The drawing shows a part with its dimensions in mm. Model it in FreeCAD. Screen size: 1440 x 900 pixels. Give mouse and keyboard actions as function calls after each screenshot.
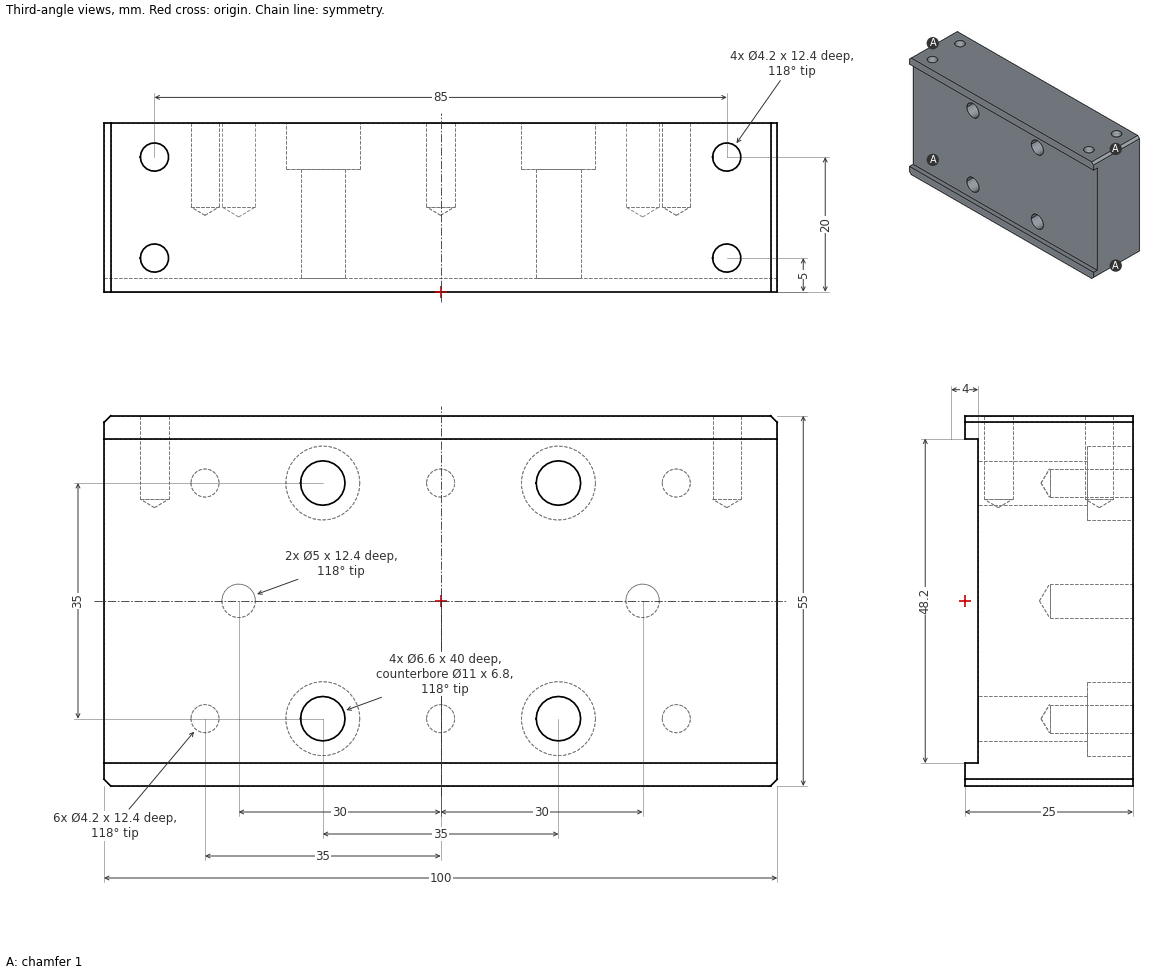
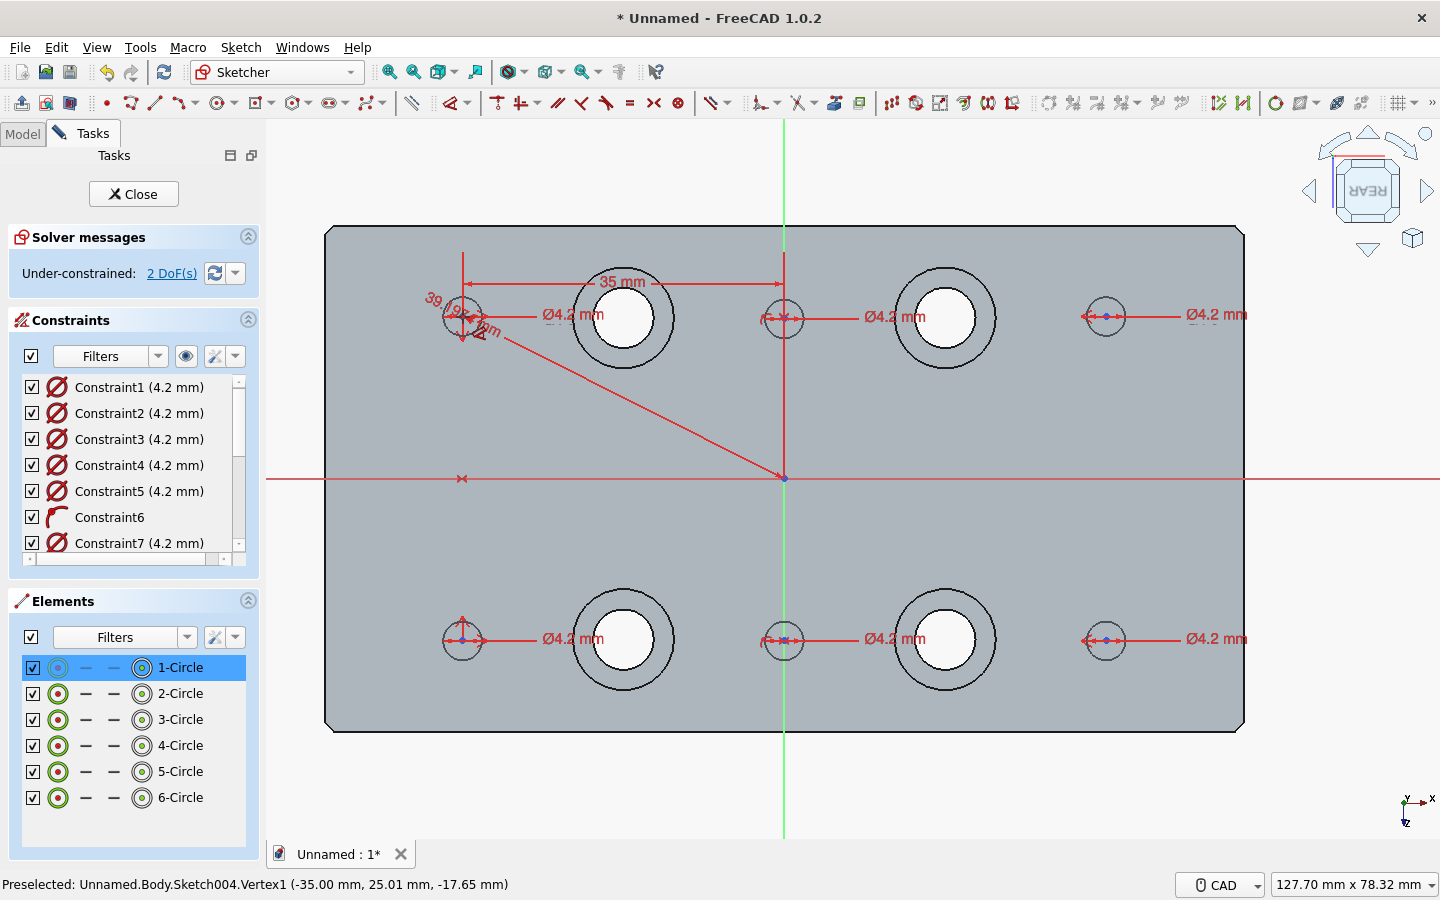
click(463, 641)
click(429, 404)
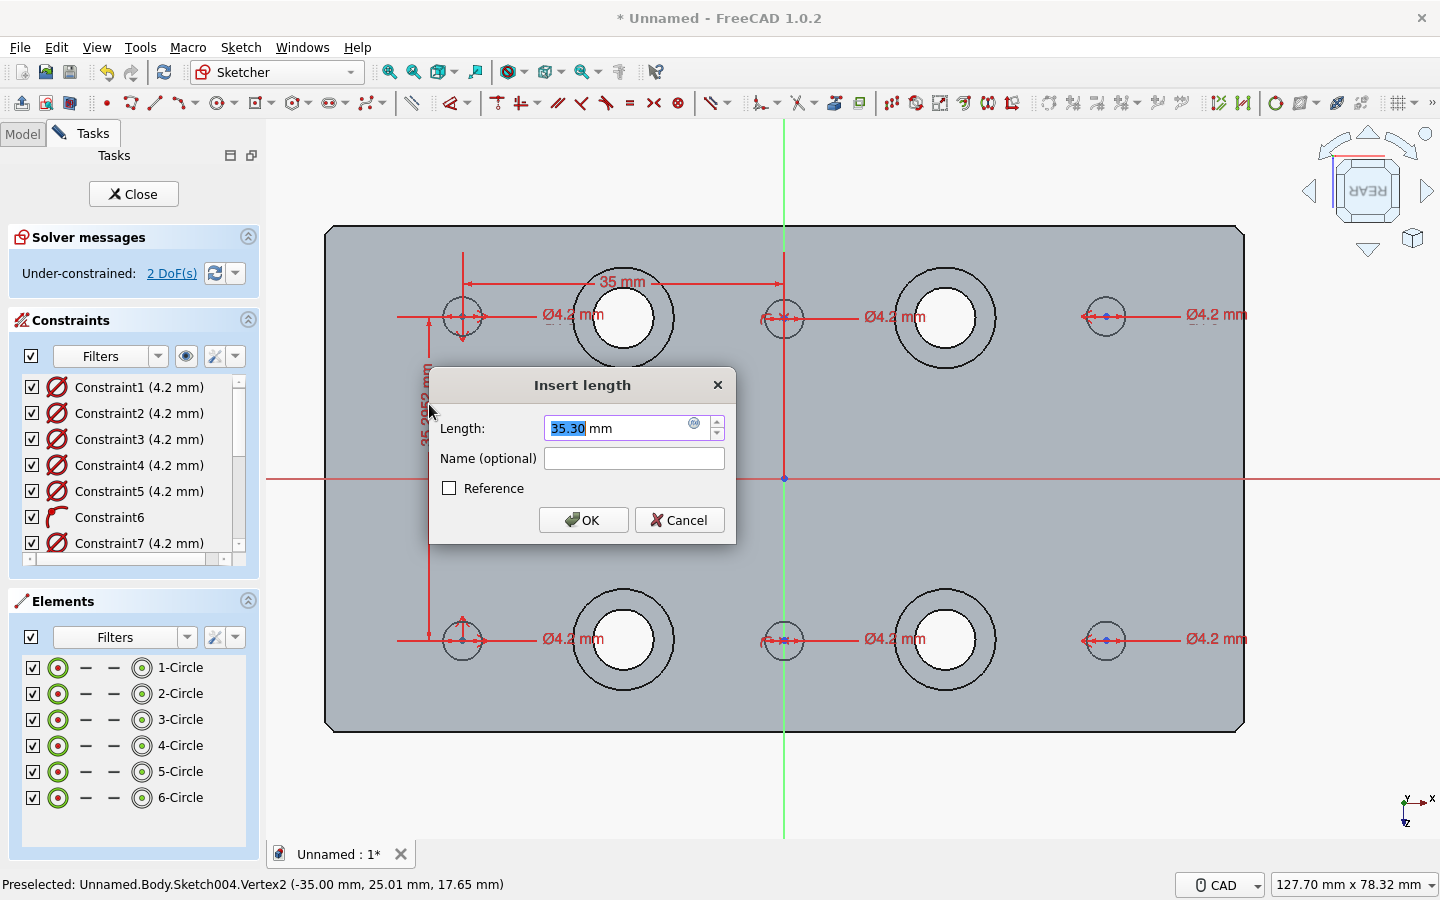
text(35)
key(Return)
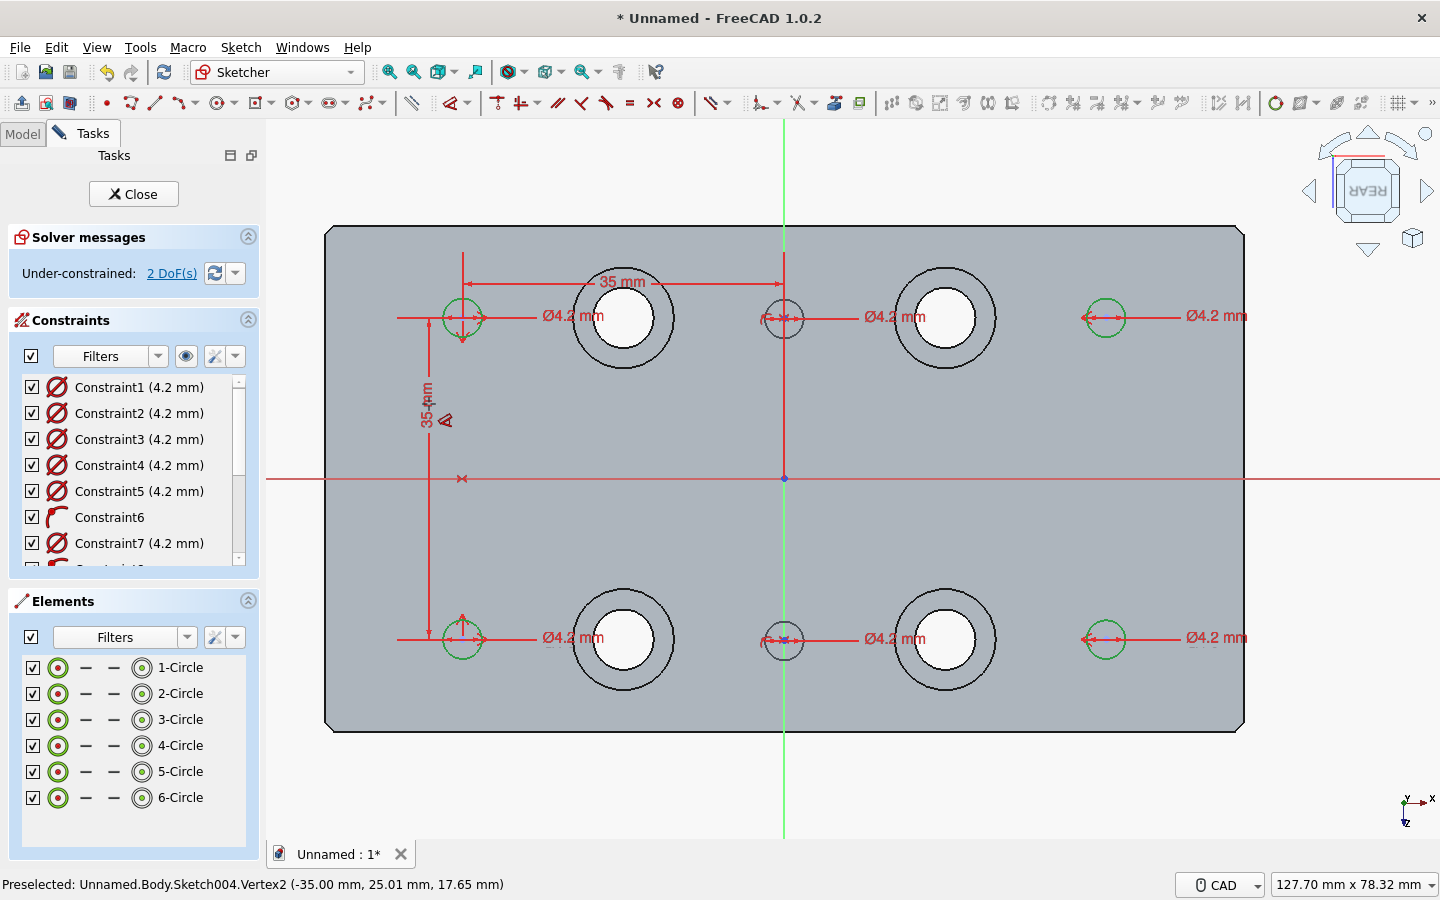
click(463, 640)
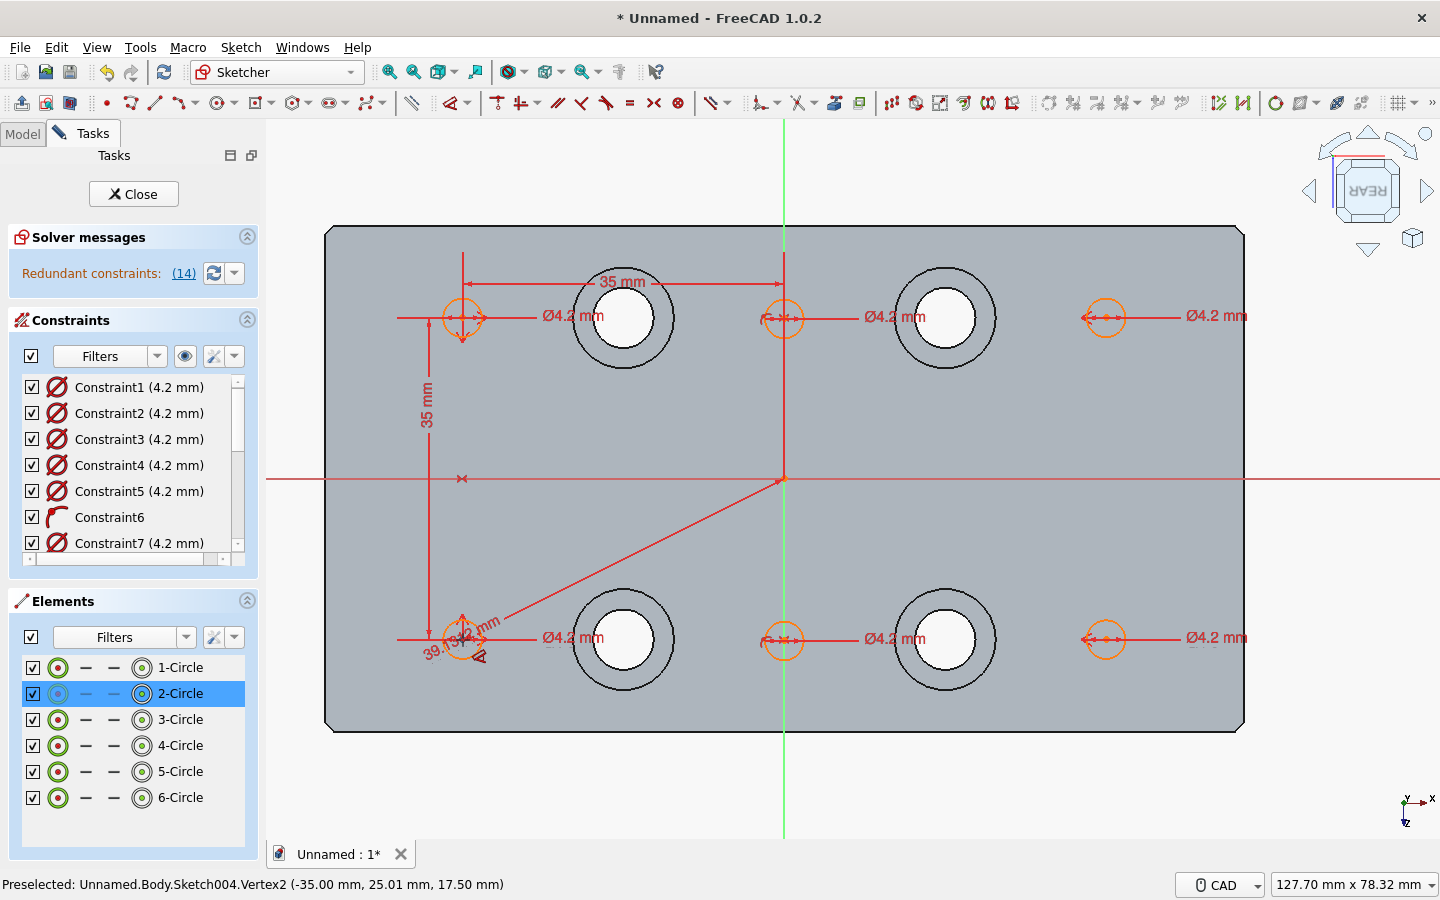
click(784, 319)
click(429, 553)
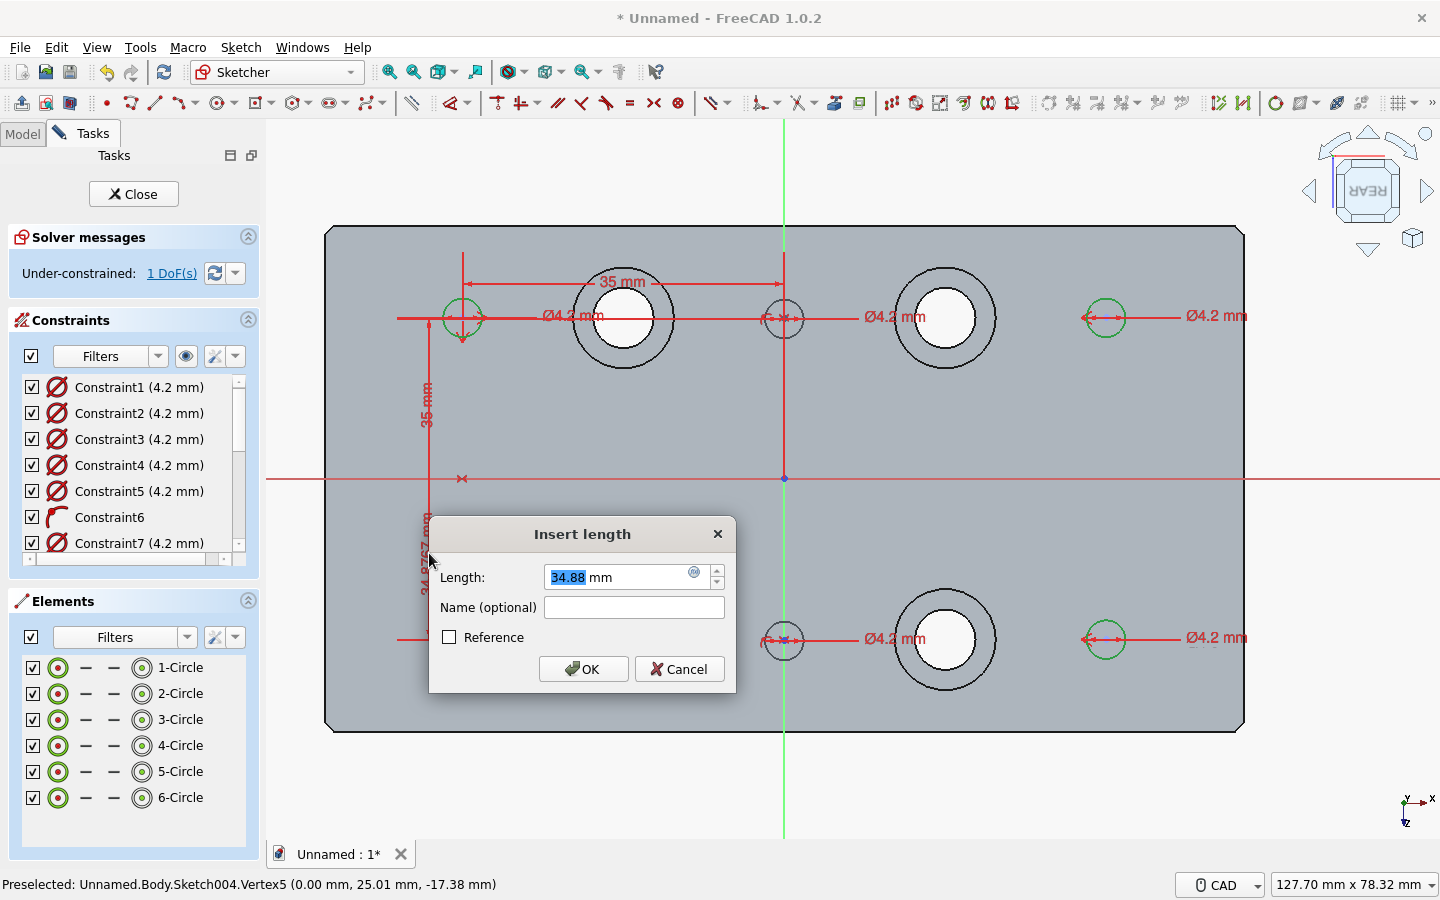
text(35)
key(Return)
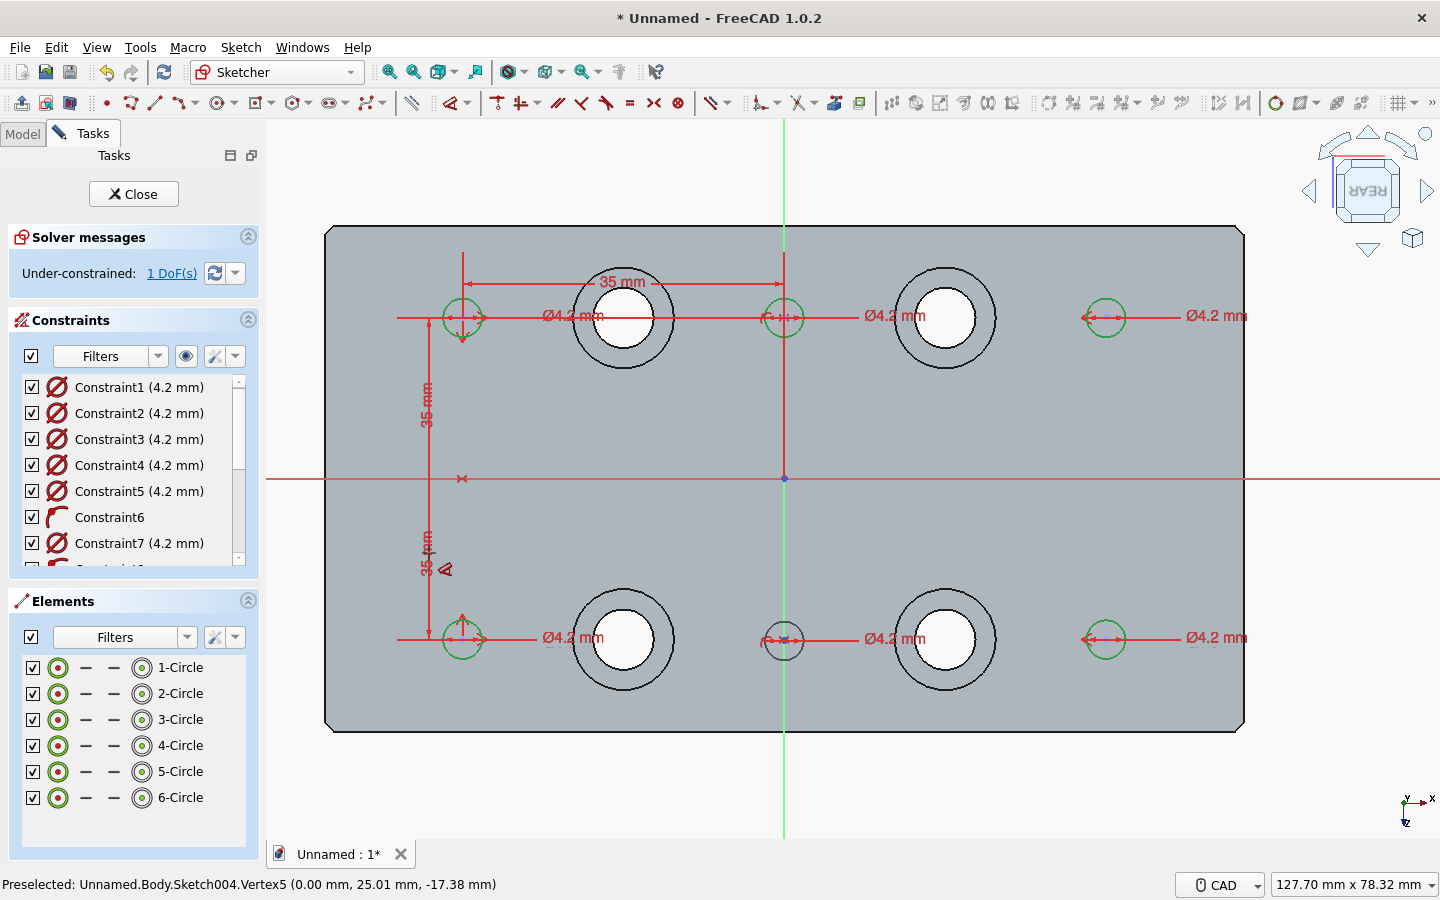
click(784, 318)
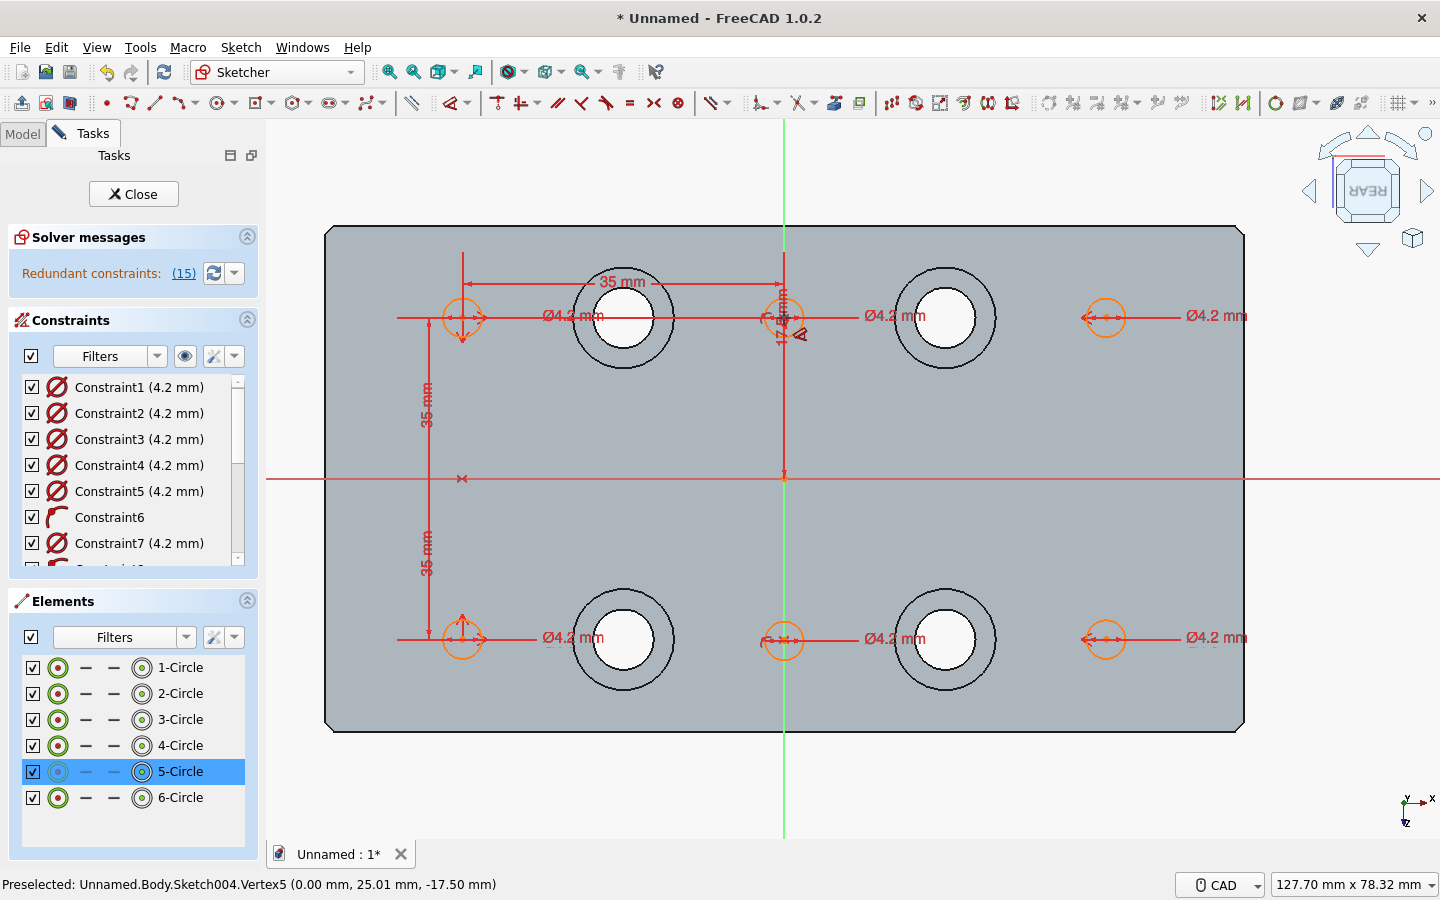
click(784, 641)
click(818, 405)